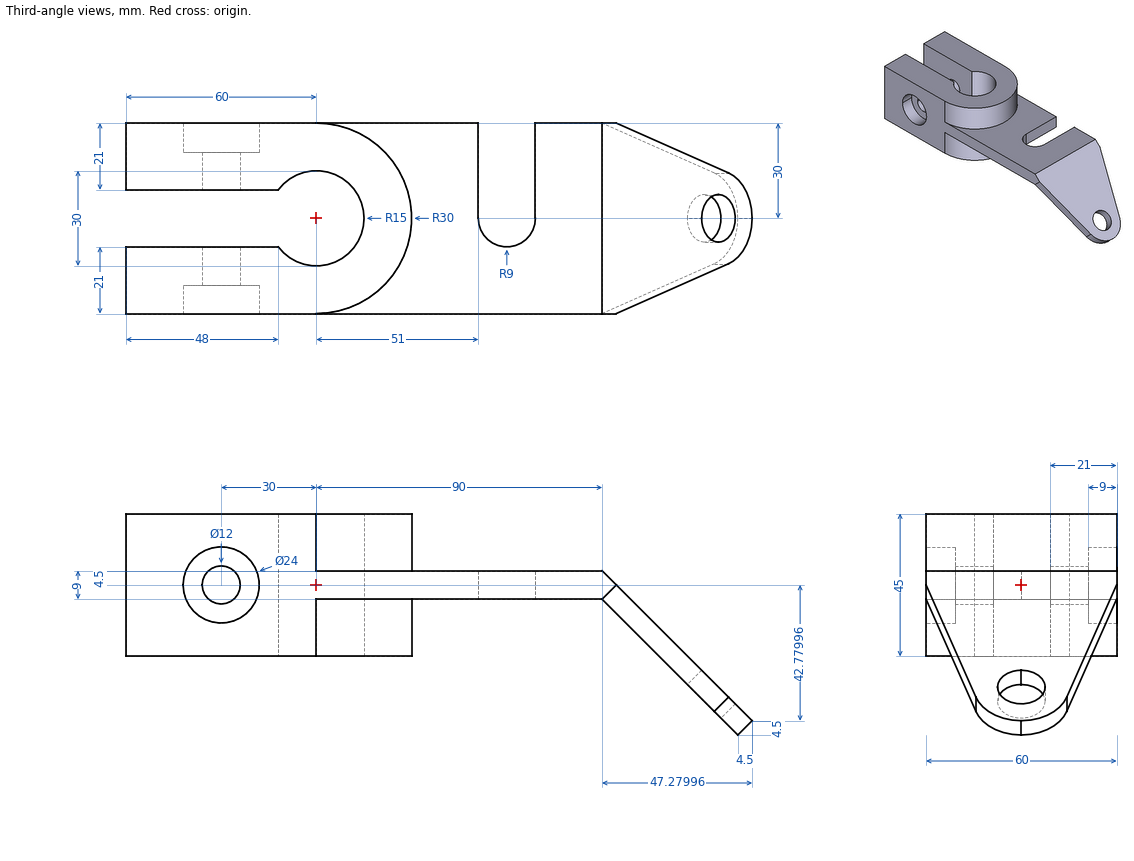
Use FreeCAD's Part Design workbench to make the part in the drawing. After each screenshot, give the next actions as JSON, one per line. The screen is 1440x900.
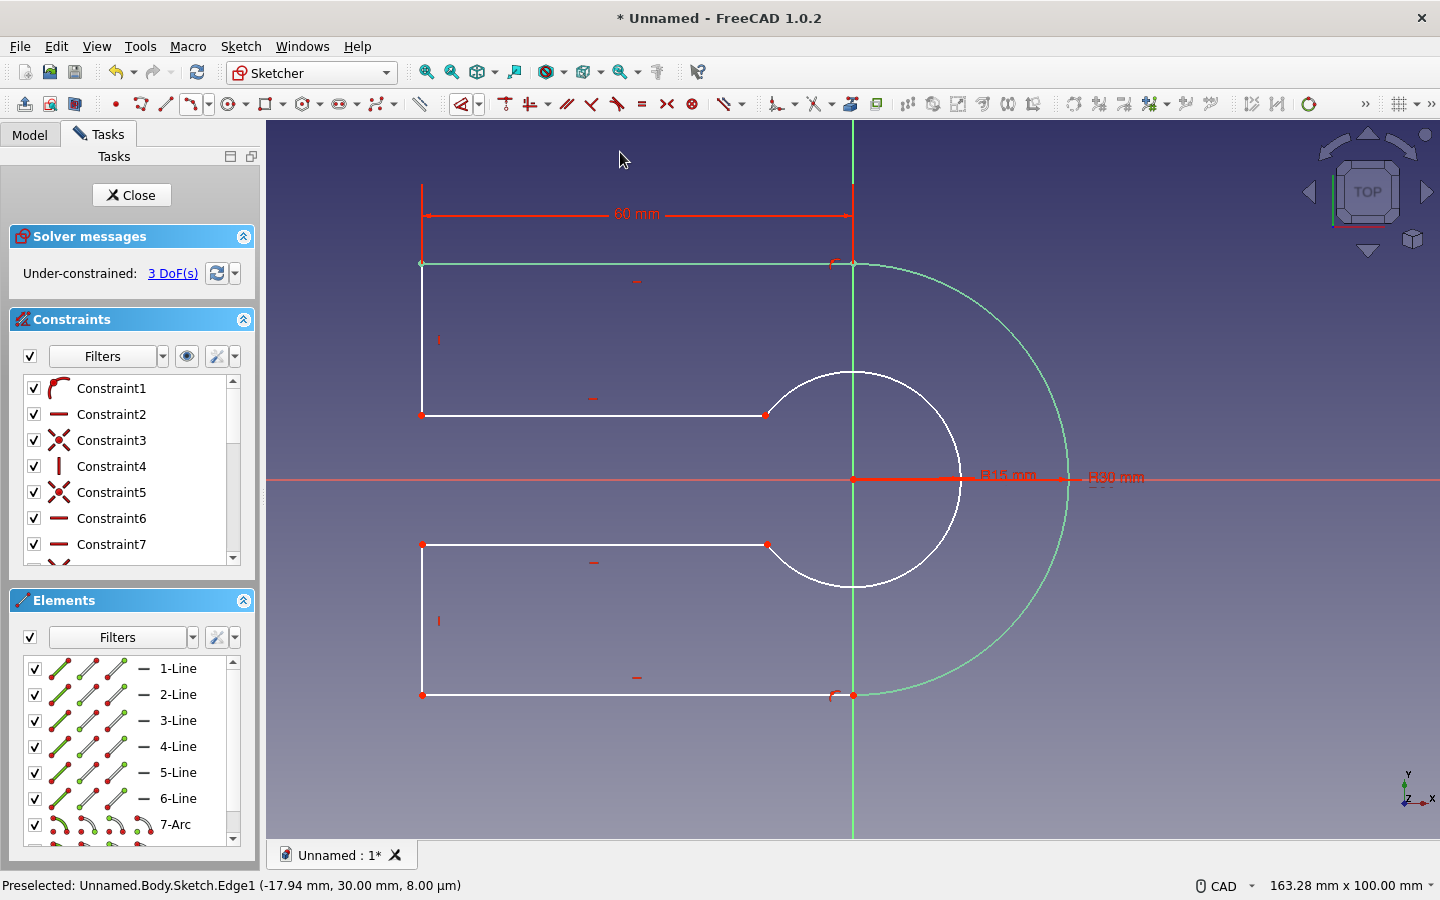
{"action": "left_click", "coordinate": [422, 309]}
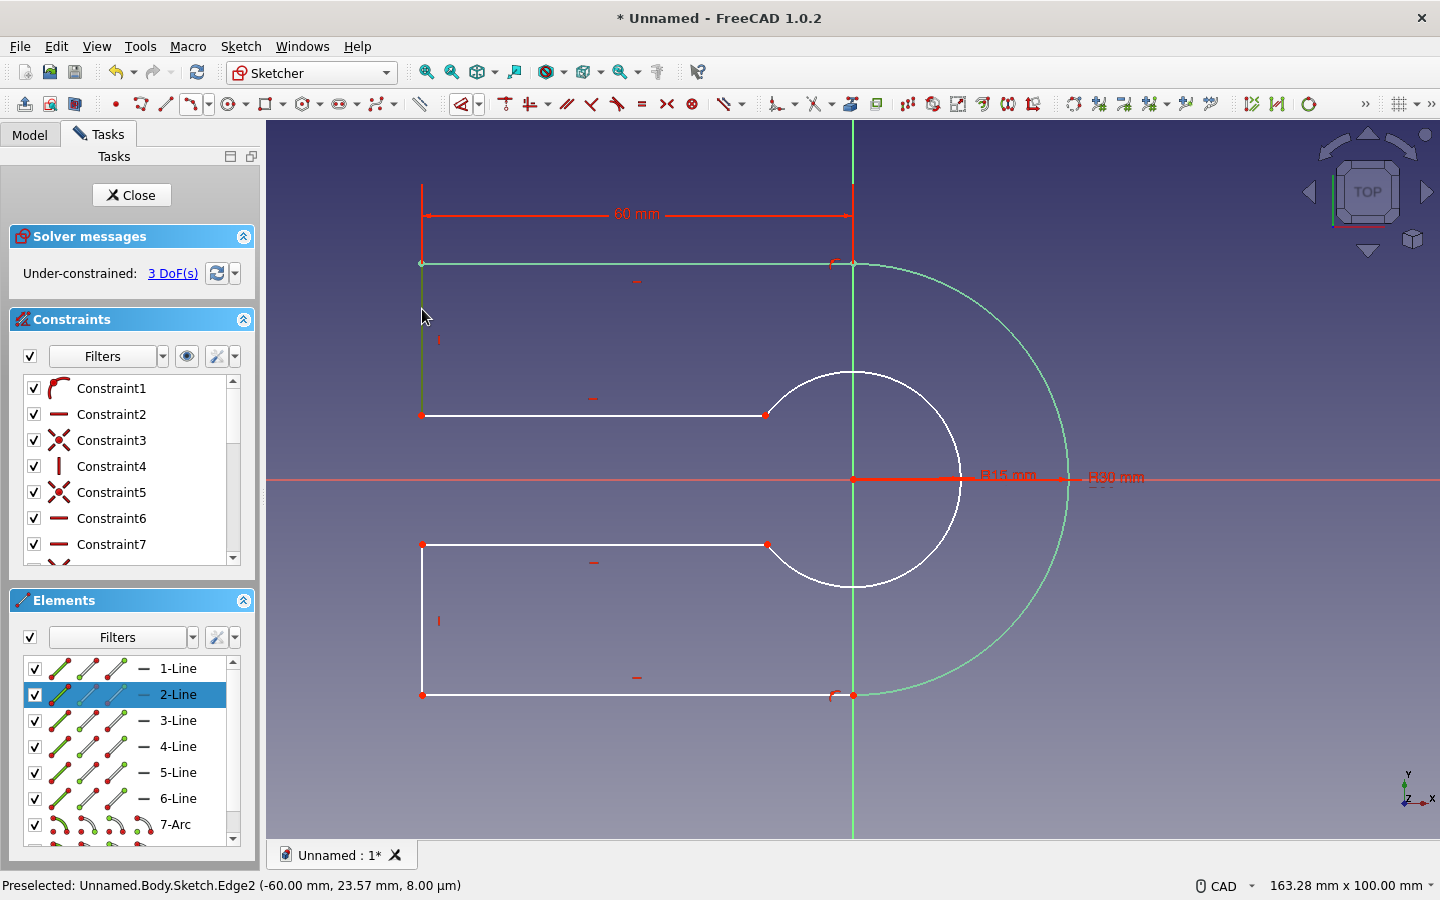
{"action": "key", "text": "i"}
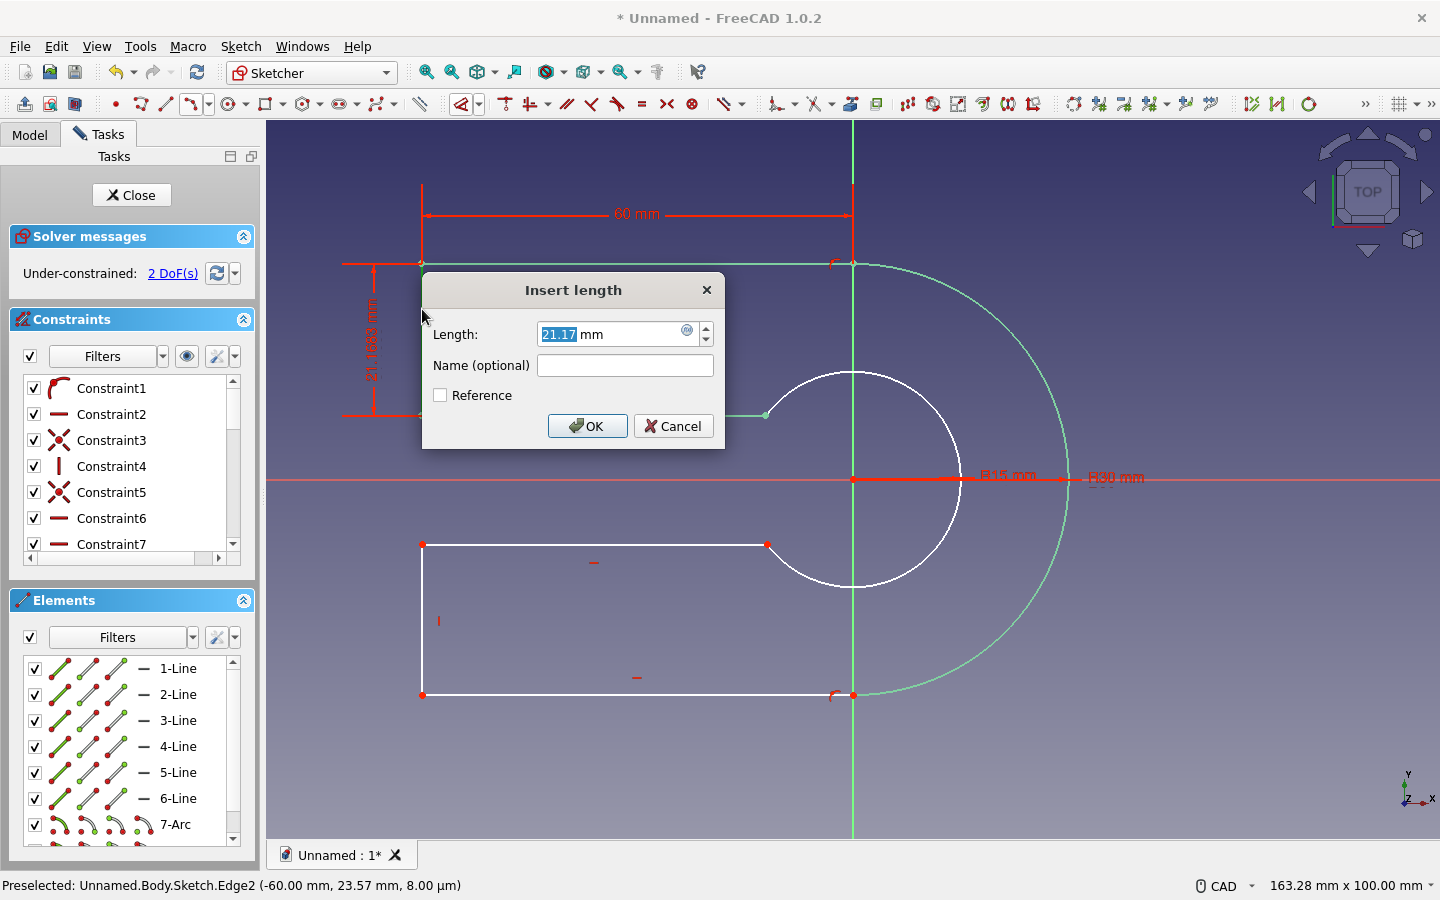
{"action": "type", "text": "21"}
{"action": "key", "text": "Return"}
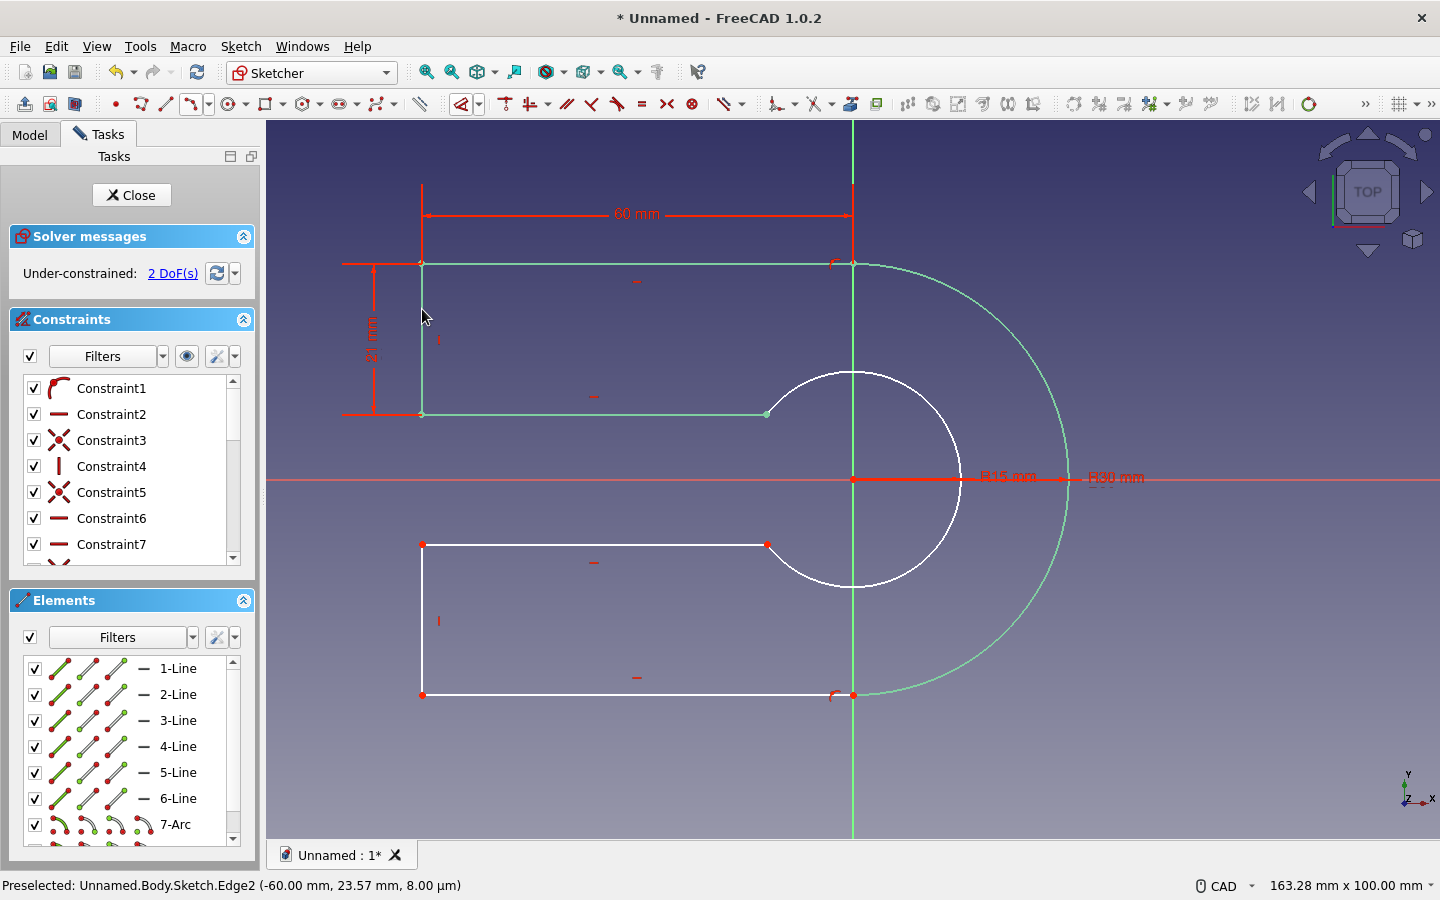
{"action": "left_click", "coordinate": [664, 545]}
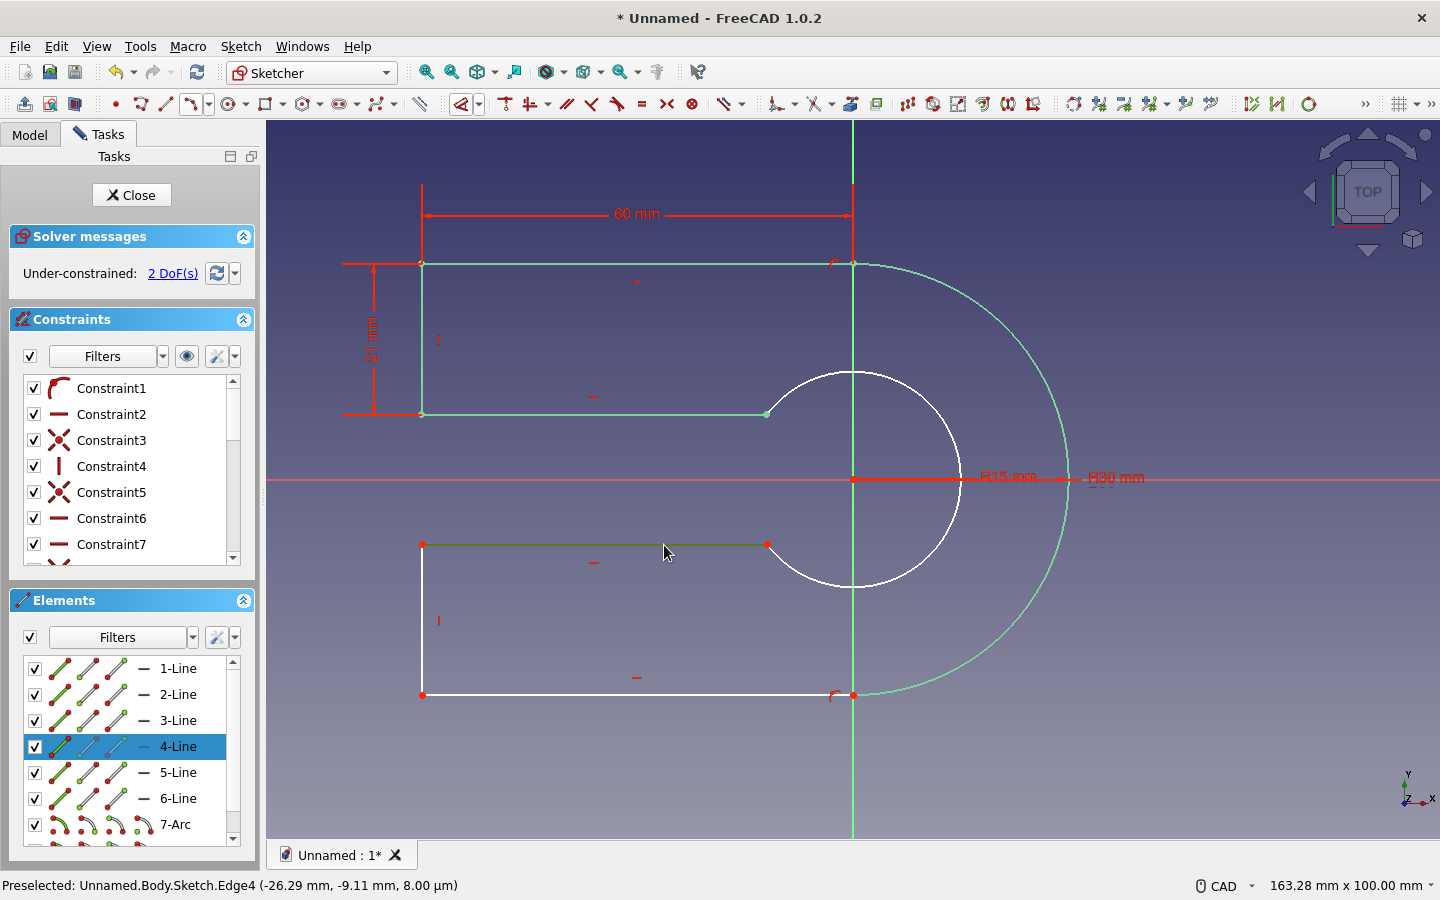
{"action": "key", "text": "l"}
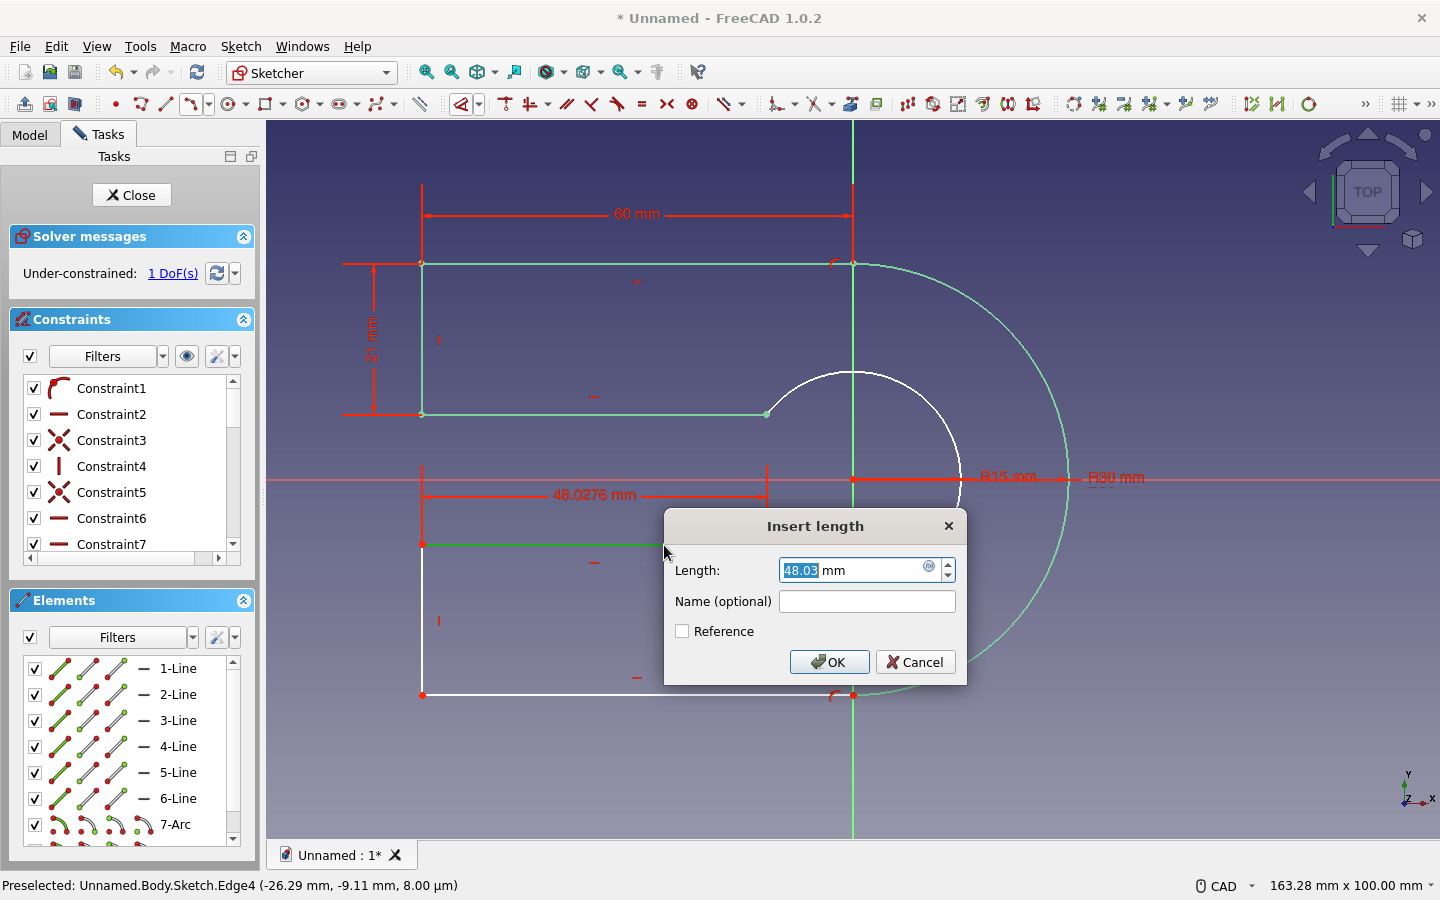
{"action": "type", "text": "48"}
{"action": "key", "text": "Return"}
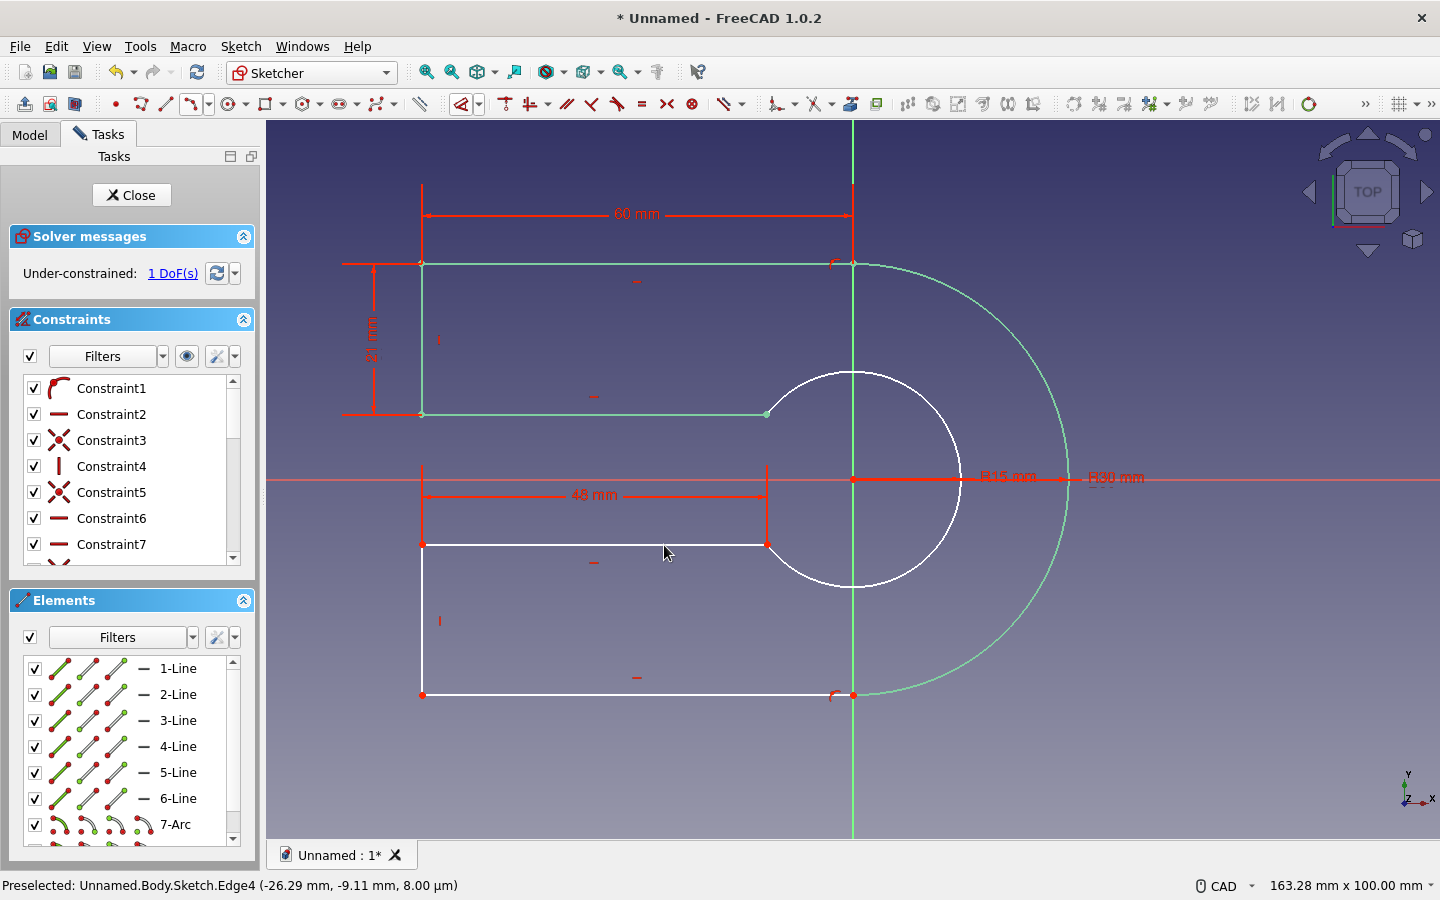
{"action": "left_click", "coordinate": [422, 590]}